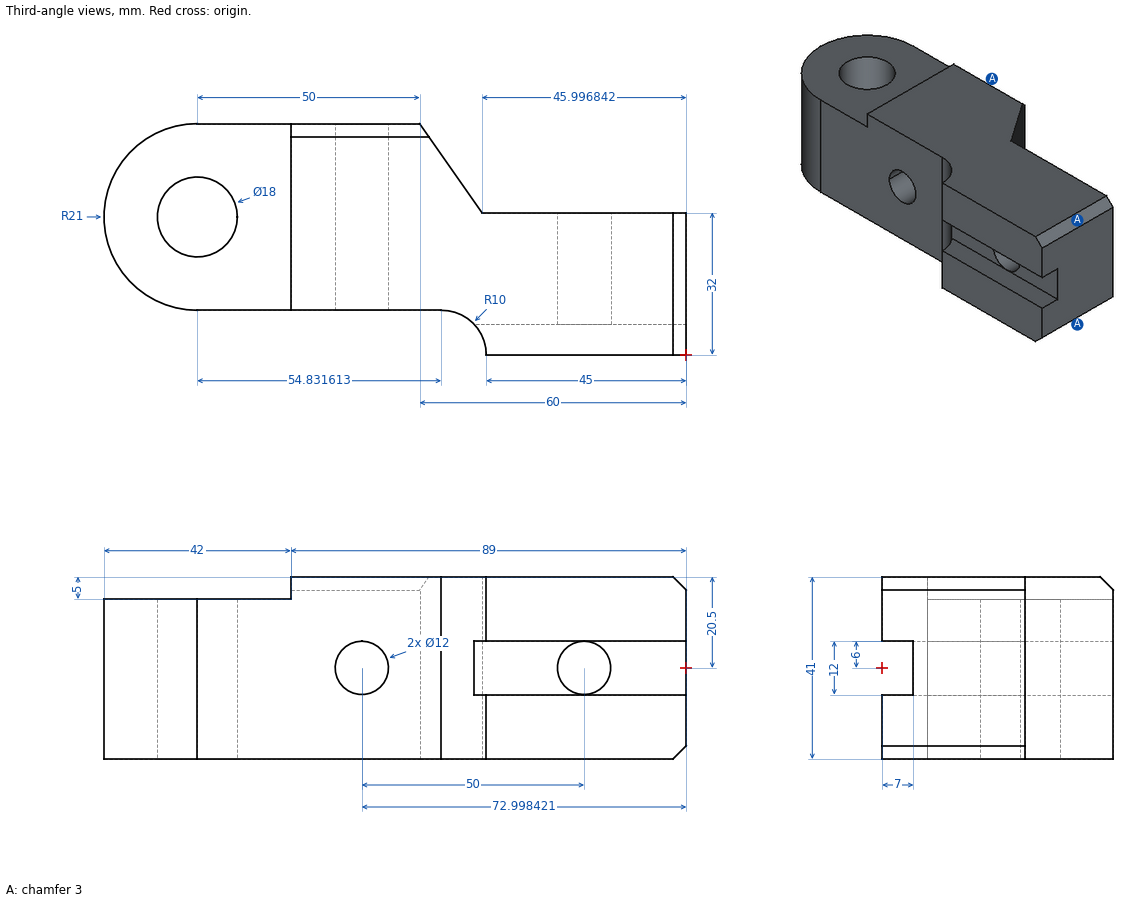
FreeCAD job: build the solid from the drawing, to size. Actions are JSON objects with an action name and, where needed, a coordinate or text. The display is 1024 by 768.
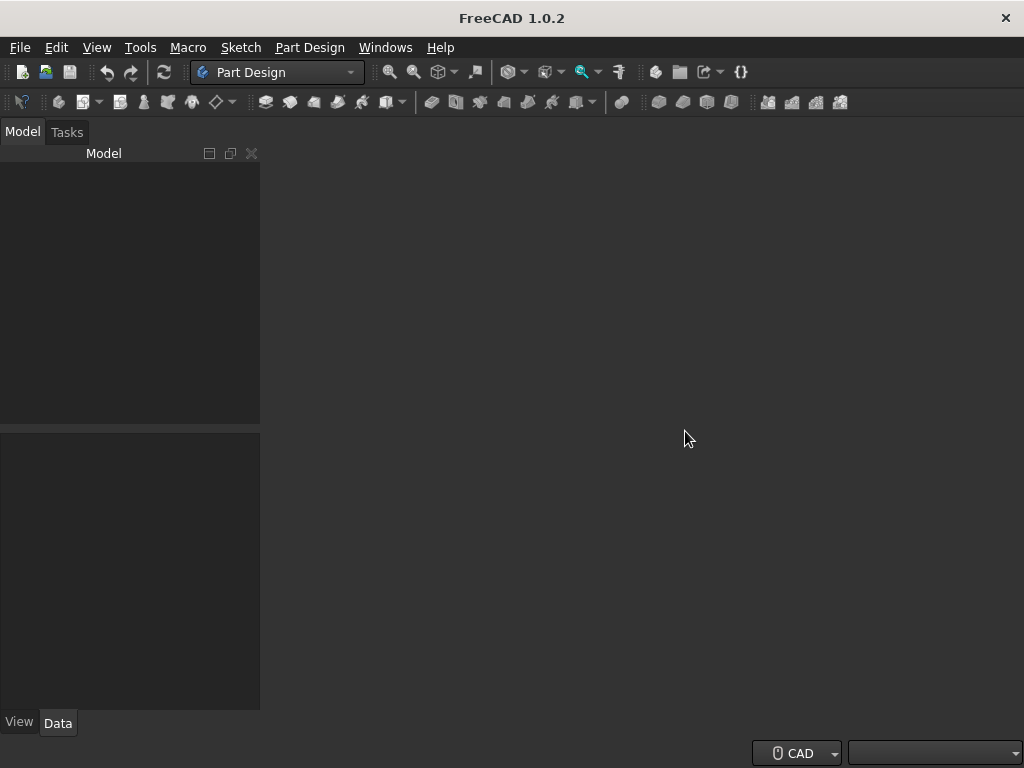
{"action": "left_click", "coordinate": [22, 72]}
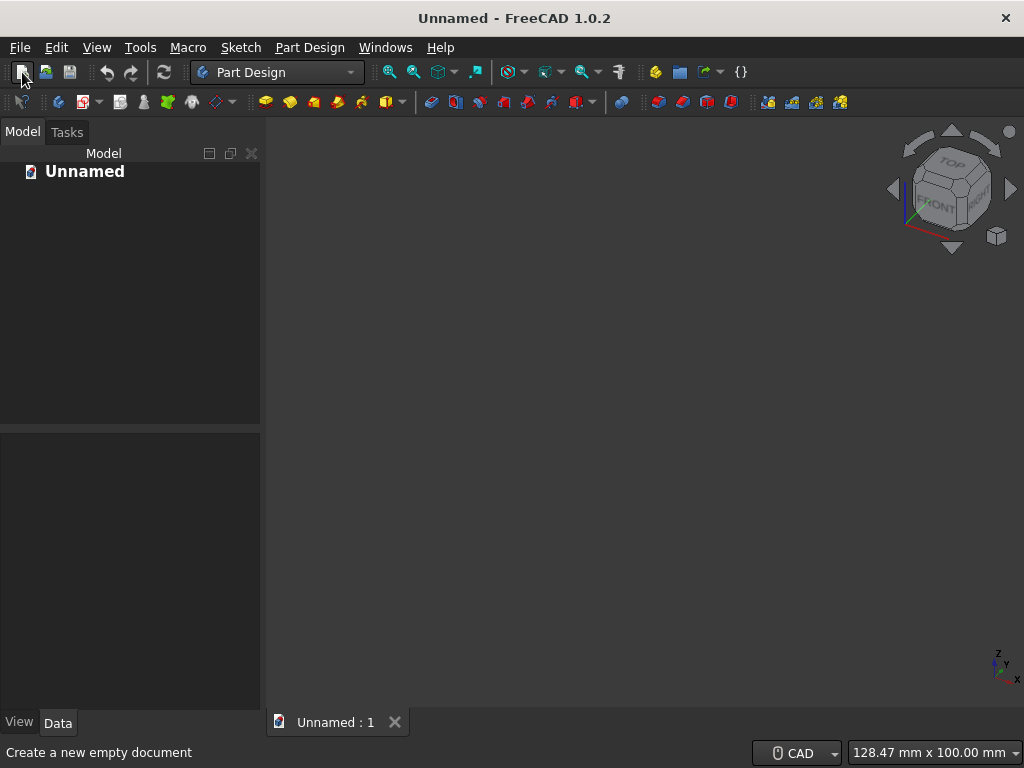
{"action": "left_click", "coordinate": [84, 102]}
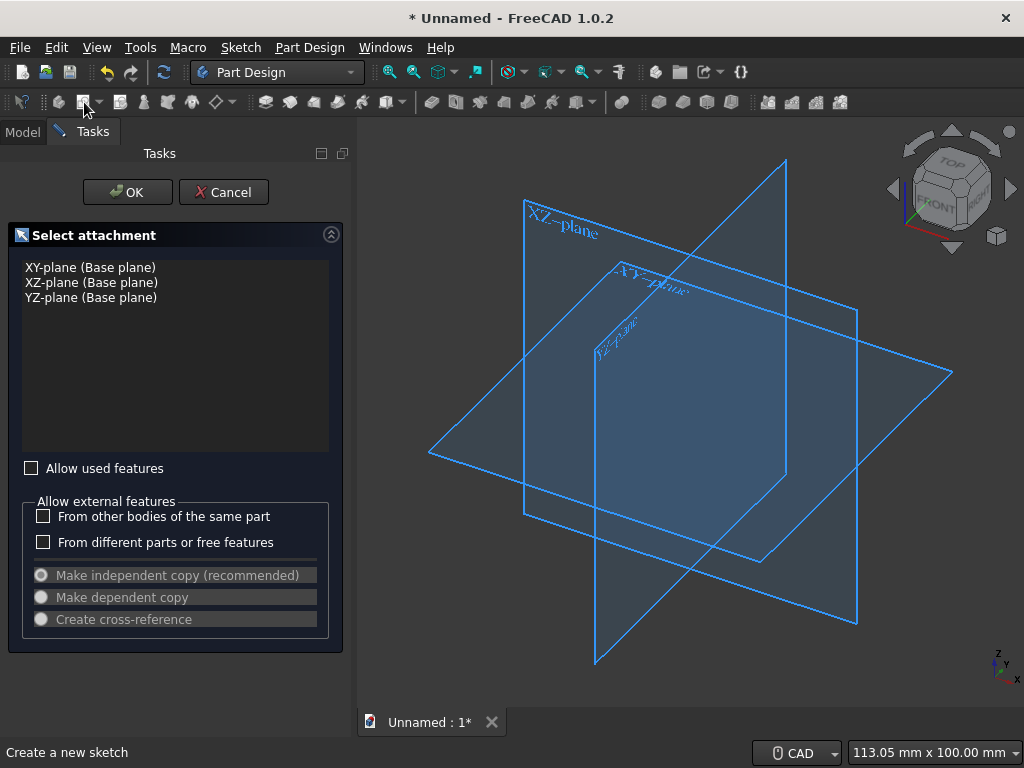
{"action": "left_click", "coordinate": [82, 268]}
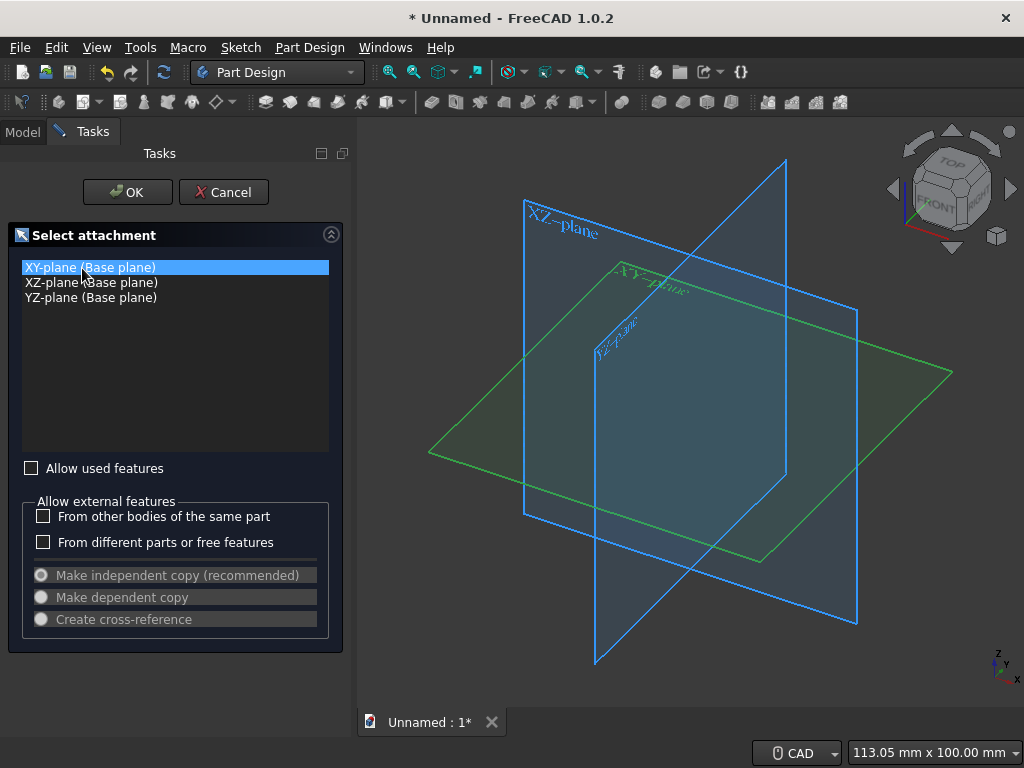
{"action": "left_click", "coordinate": [128, 192]}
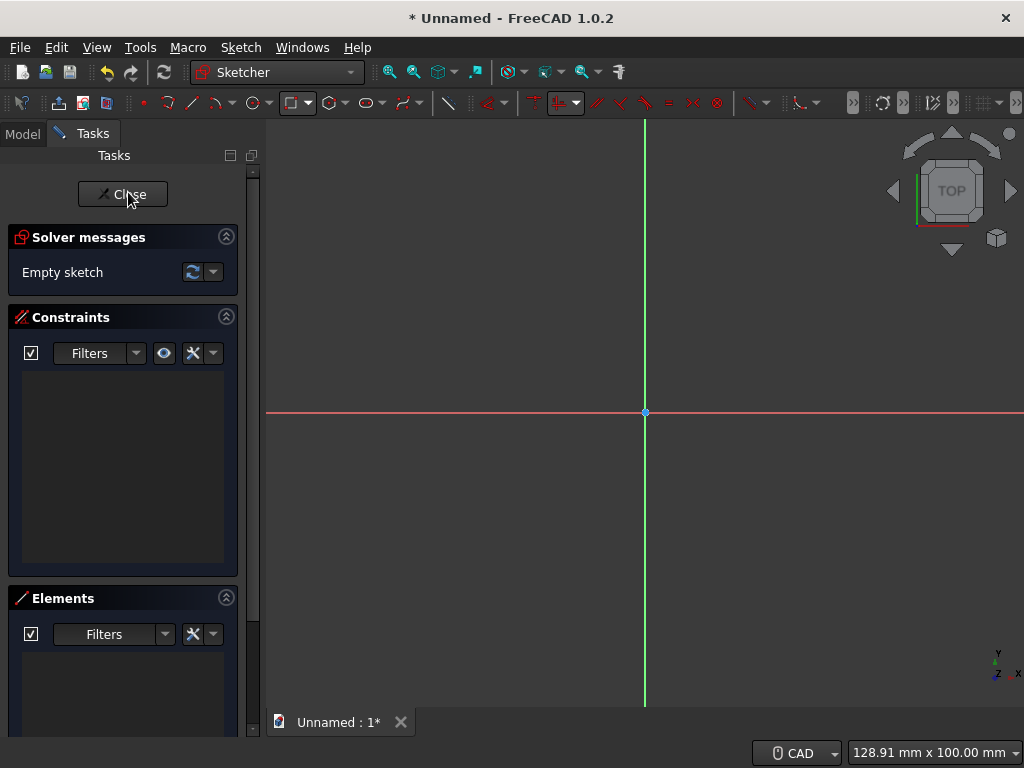
{"action": "scroll", "coordinate": [835, 538], "scroll_direction": "down", "scroll_amount": 4}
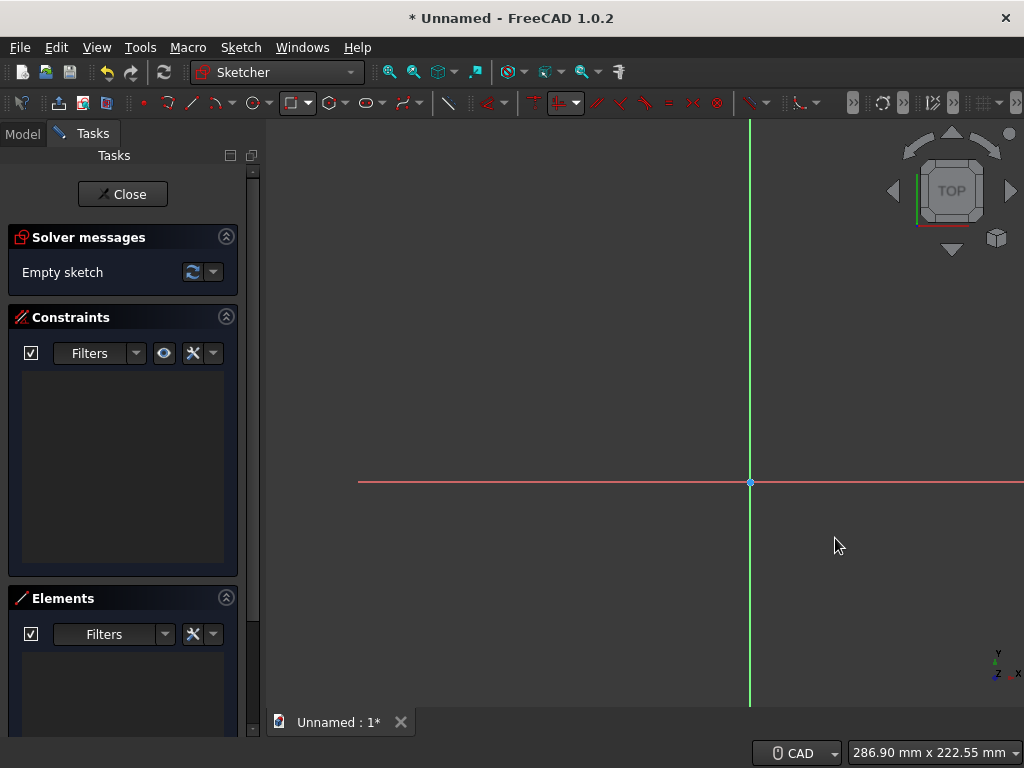
{"action": "left_click", "coordinate": [168, 104]}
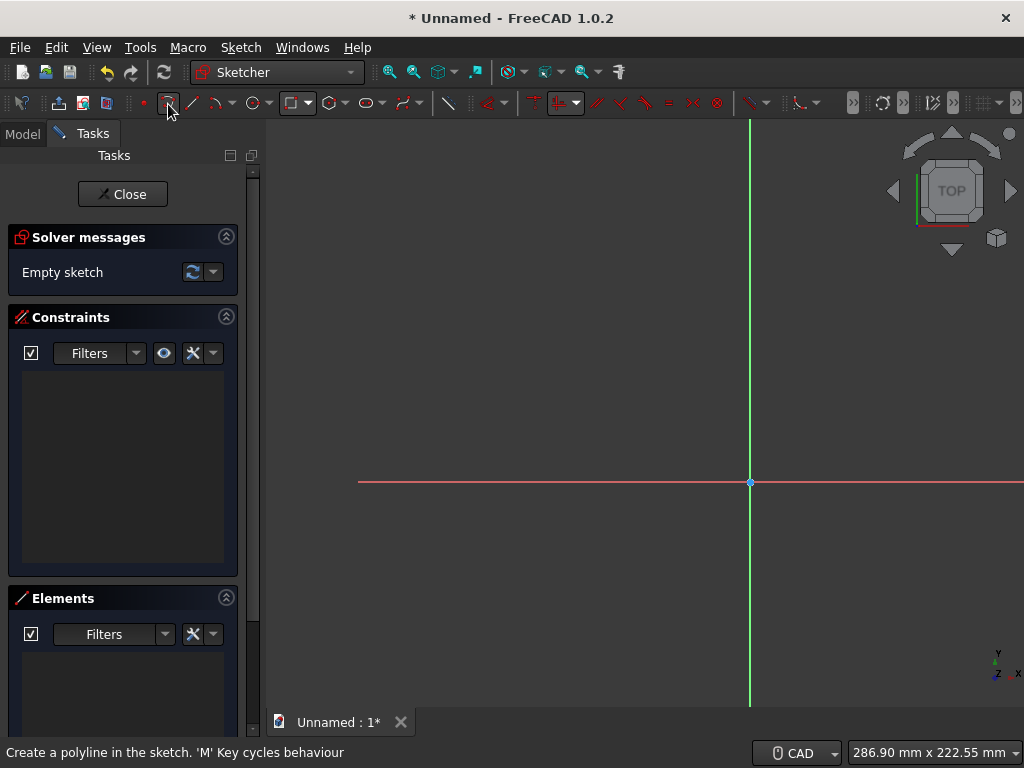
{"action": "left_click", "coordinate": [631, 482]}
{"action": "left_click", "coordinate": [750, 482]}
{"action": "left_click", "coordinate": [741, 398]}
{"action": "left_click", "coordinate": [629, 398]}
{"action": "left_click", "coordinate": [592, 345]}
{"action": "left_click", "coordinate": [459, 345]}
{"action": "right_click", "coordinate": [459, 345]}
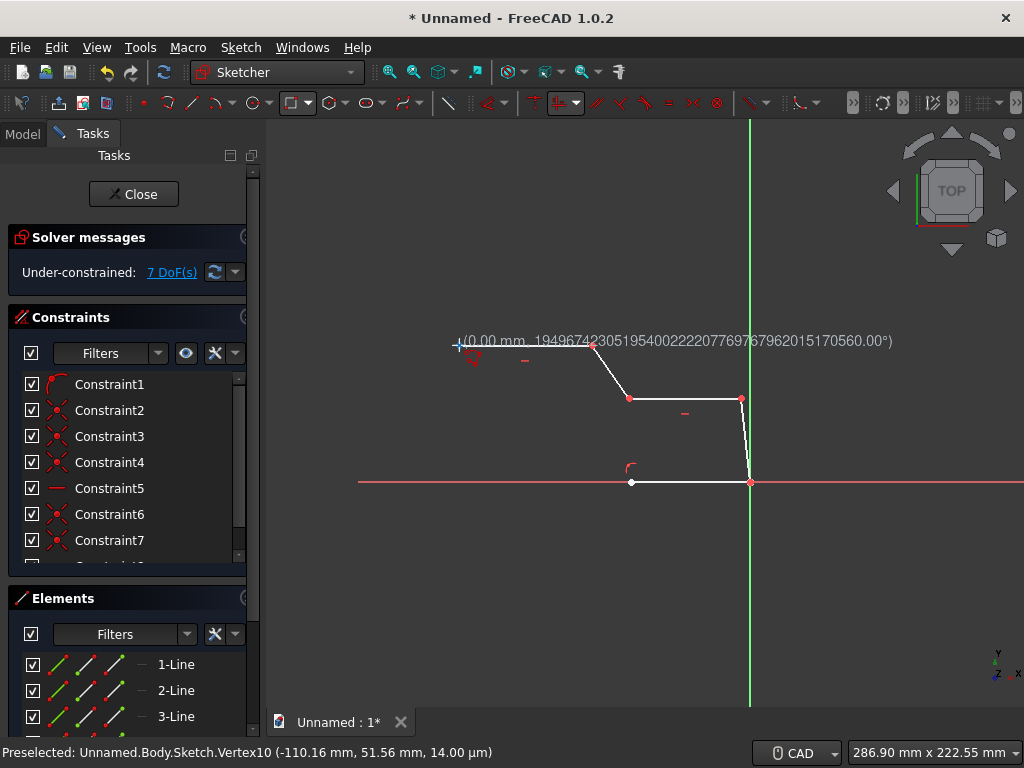
{"action": "left_click", "coordinate": [192, 104]}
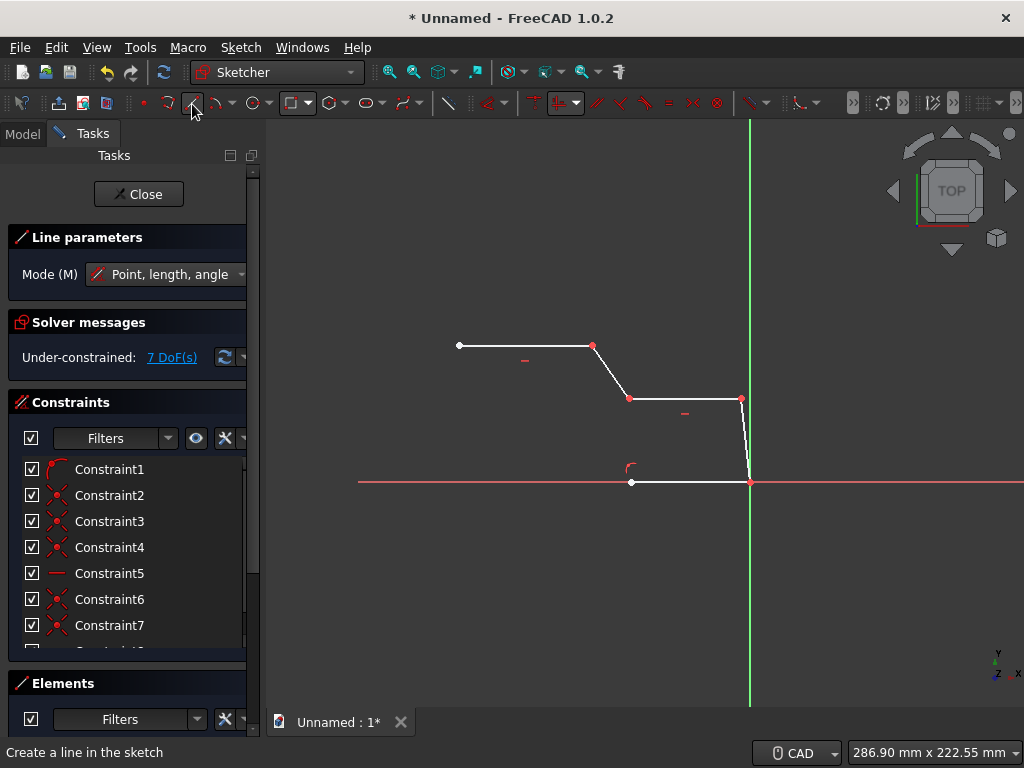
{"action": "left_click", "coordinate": [459, 456]}
{"action": "left_click", "coordinate": [604, 456]}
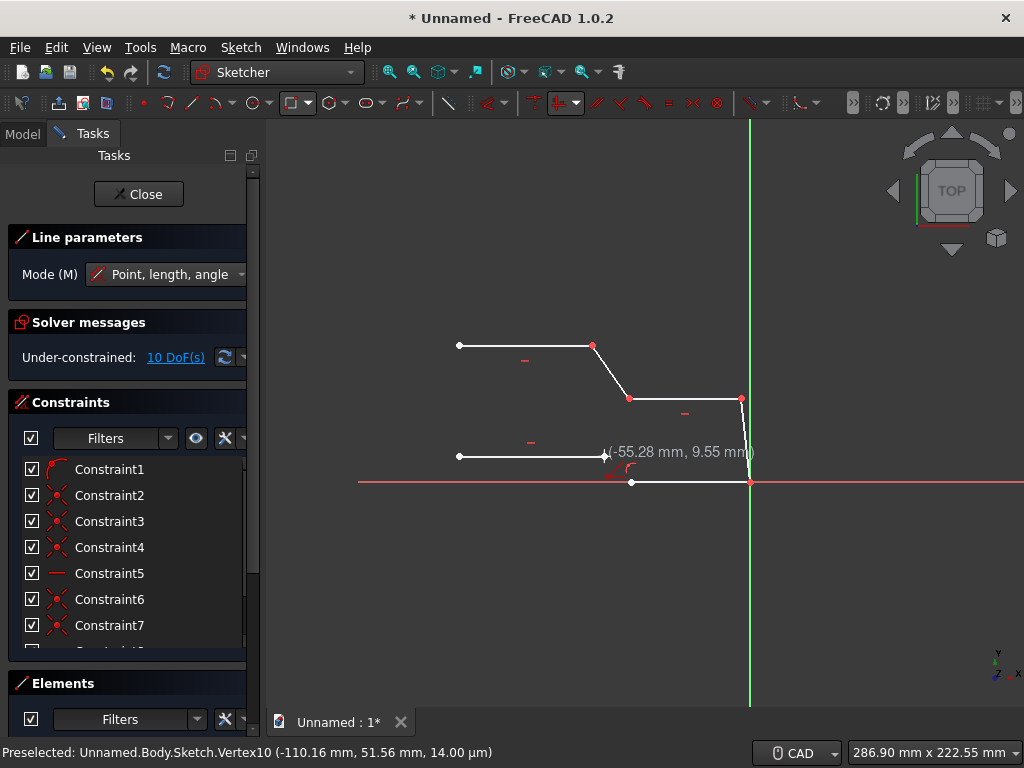
{"action": "left_click", "coordinate": [234, 104]}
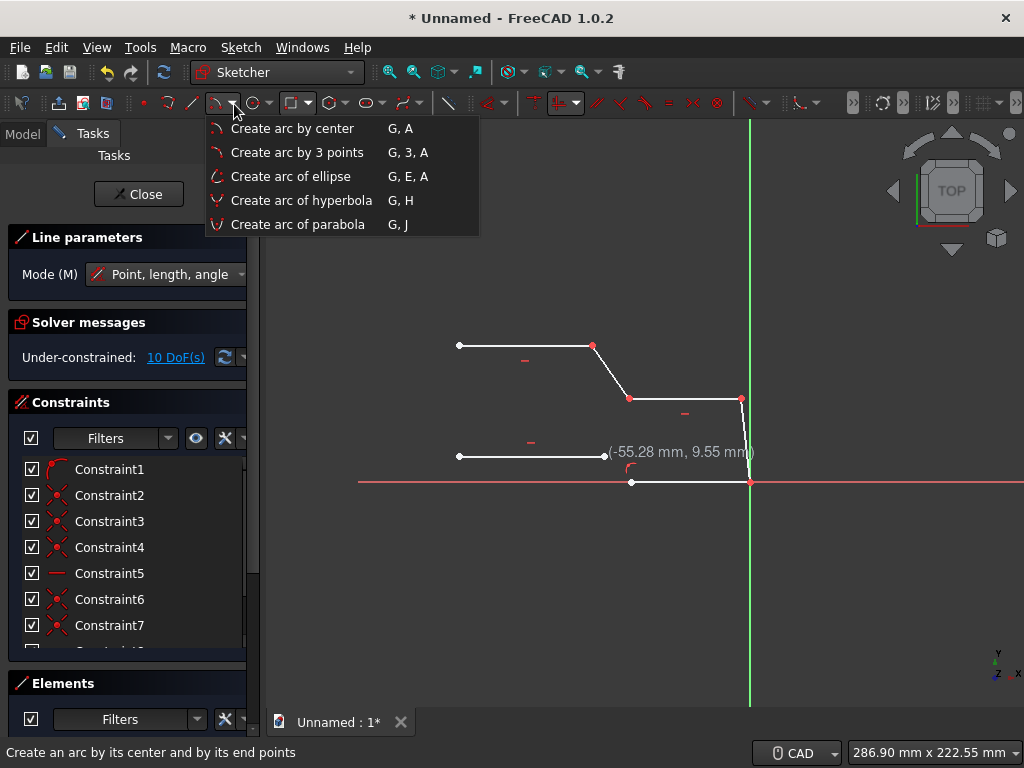
{"action": "left_click", "coordinate": [342, 152]}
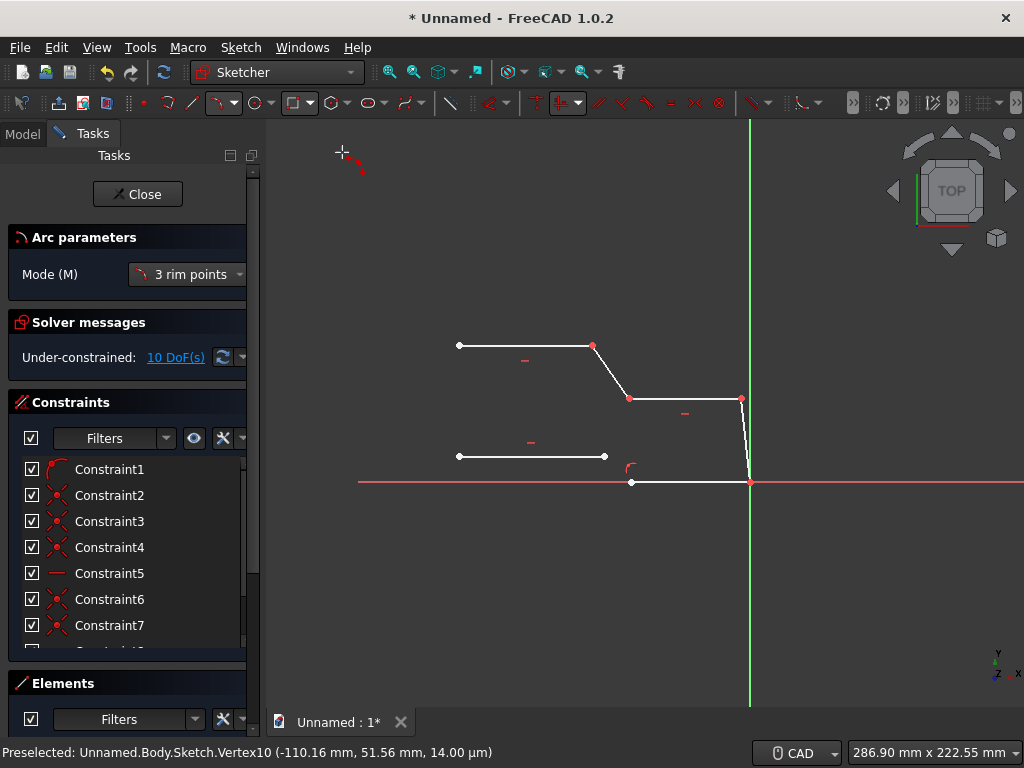
{"action": "left_click", "coordinate": [459, 346]}
{"action": "left_click", "coordinate": [459, 457]}
{"action": "left_click", "coordinate": [404, 400]}